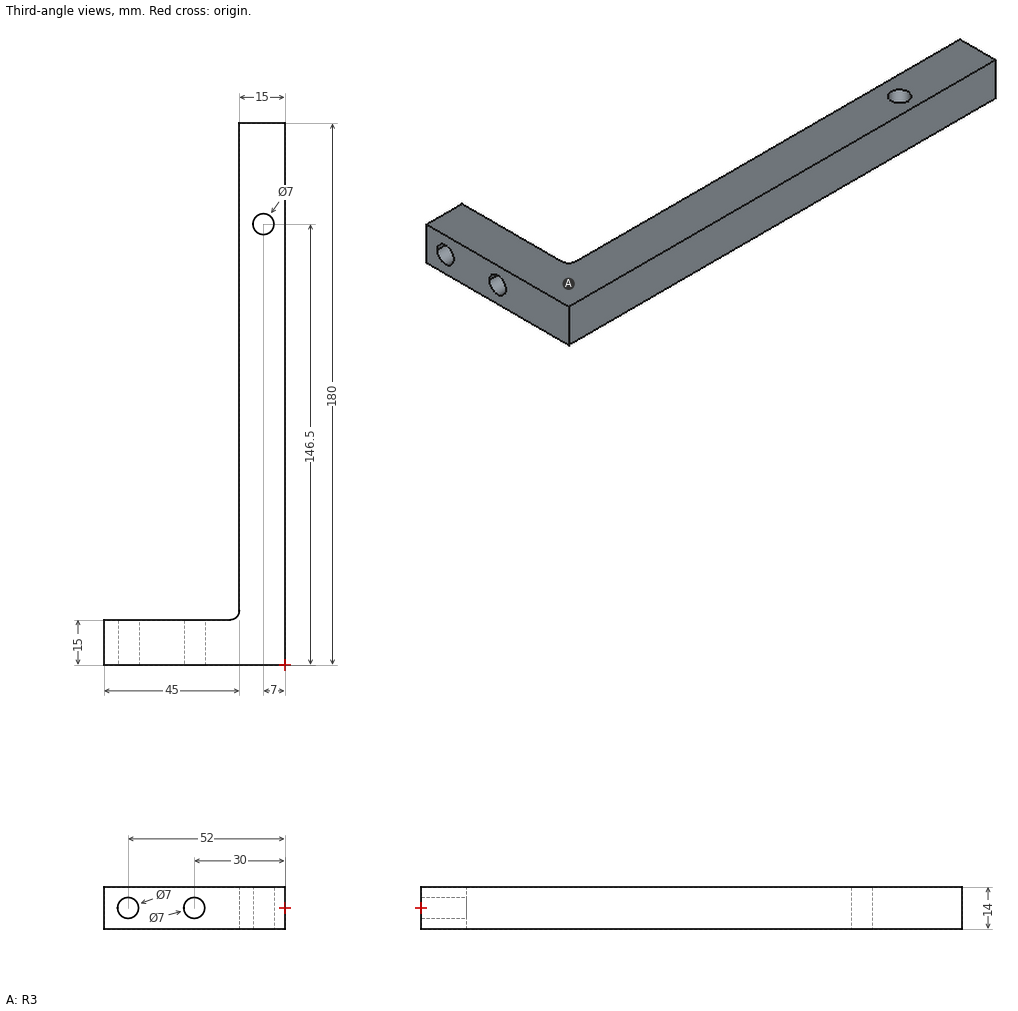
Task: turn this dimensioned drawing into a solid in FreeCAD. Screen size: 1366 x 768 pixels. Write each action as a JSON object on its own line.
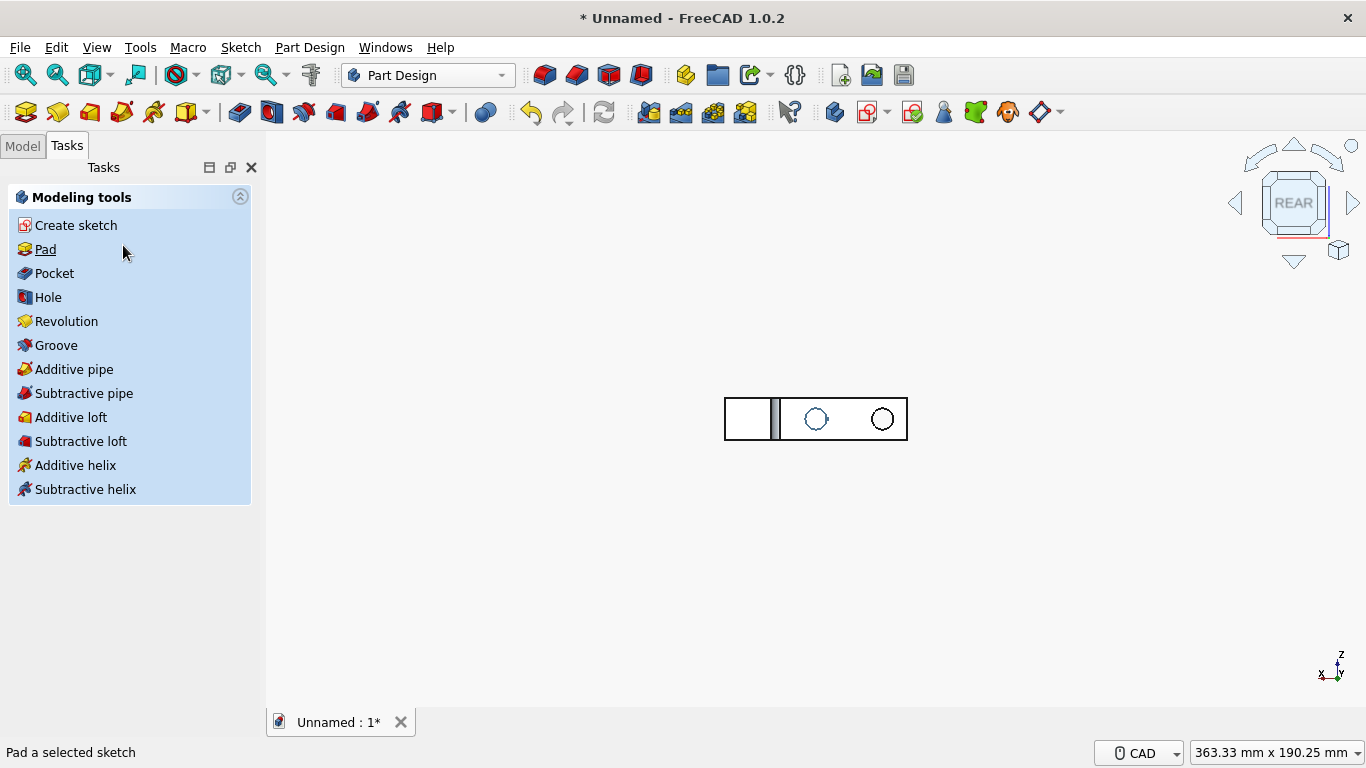
{"action": "left_click", "coordinate": [240, 112]}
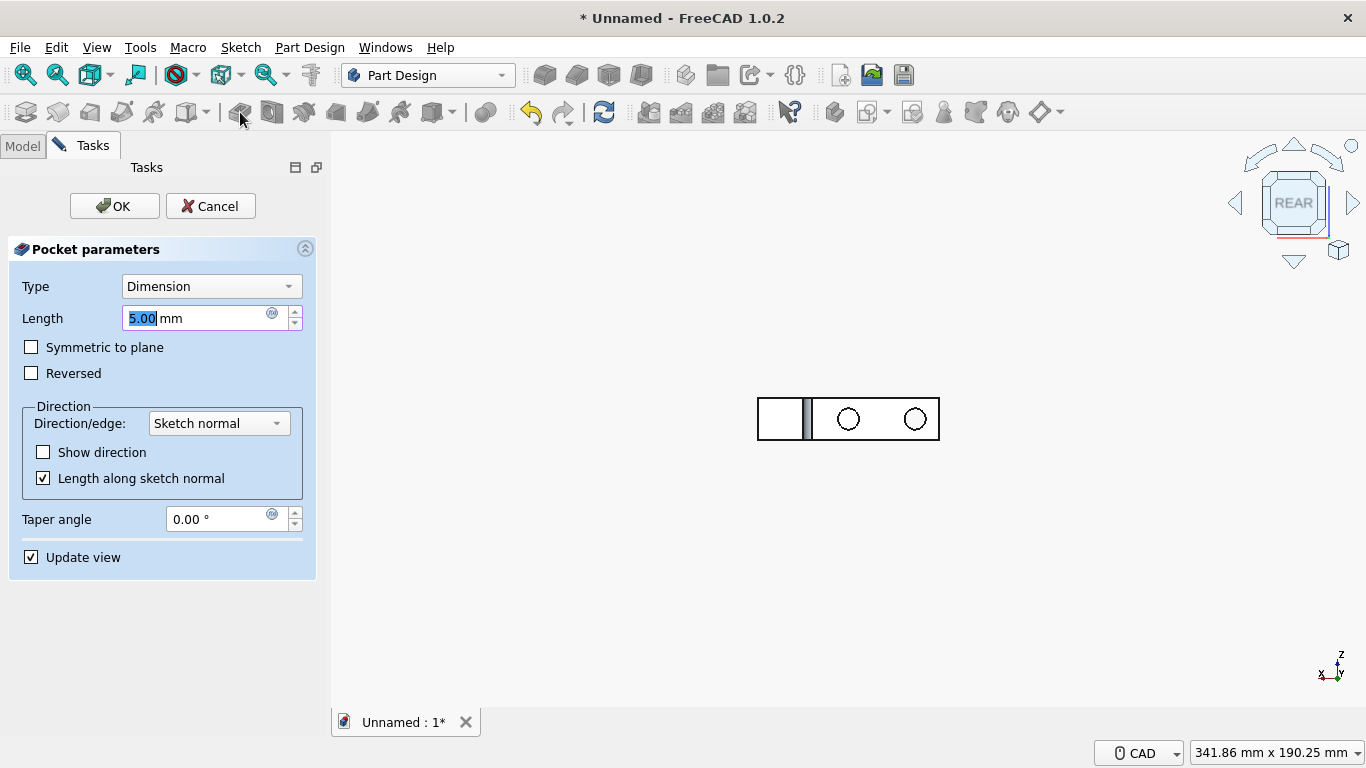
{"action": "left_click", "coordinate": [212, 286]}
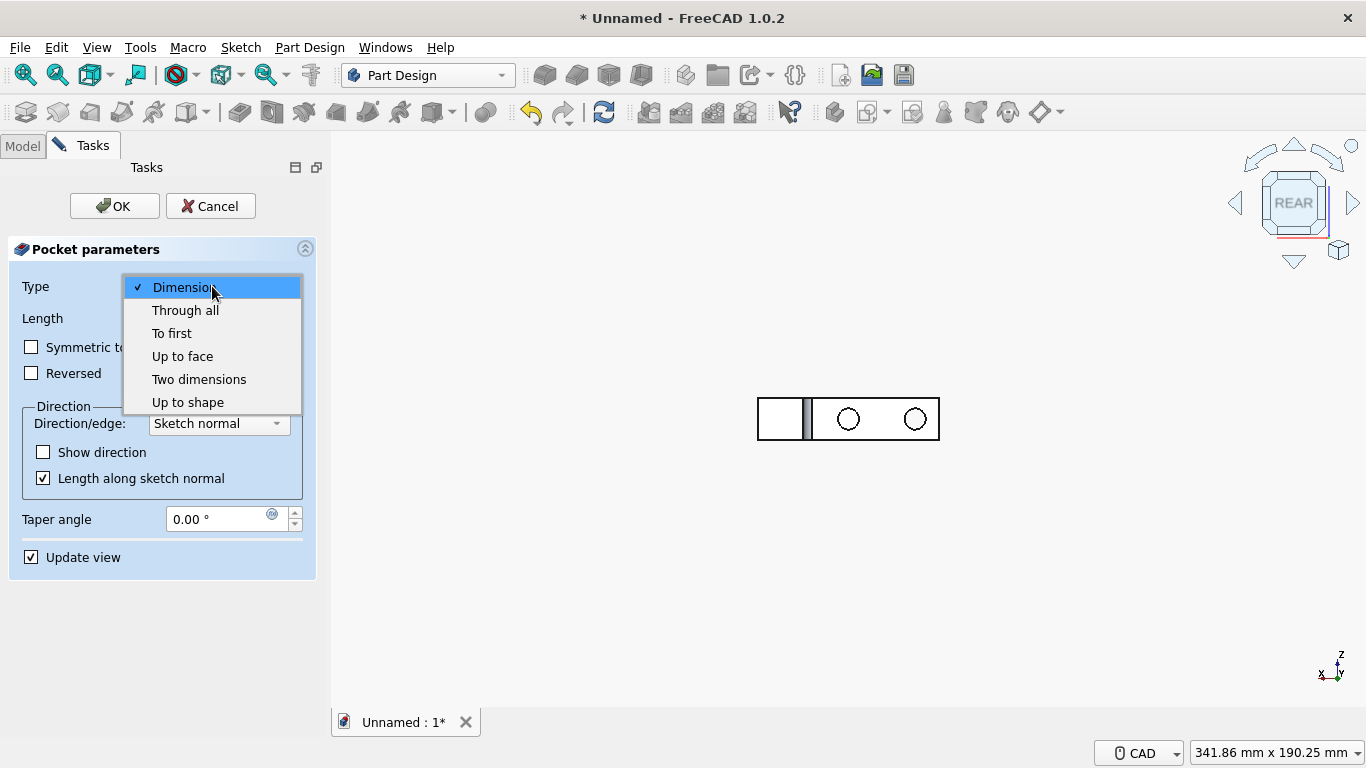
{"action": "left_click", "coordinate": [212, 334]}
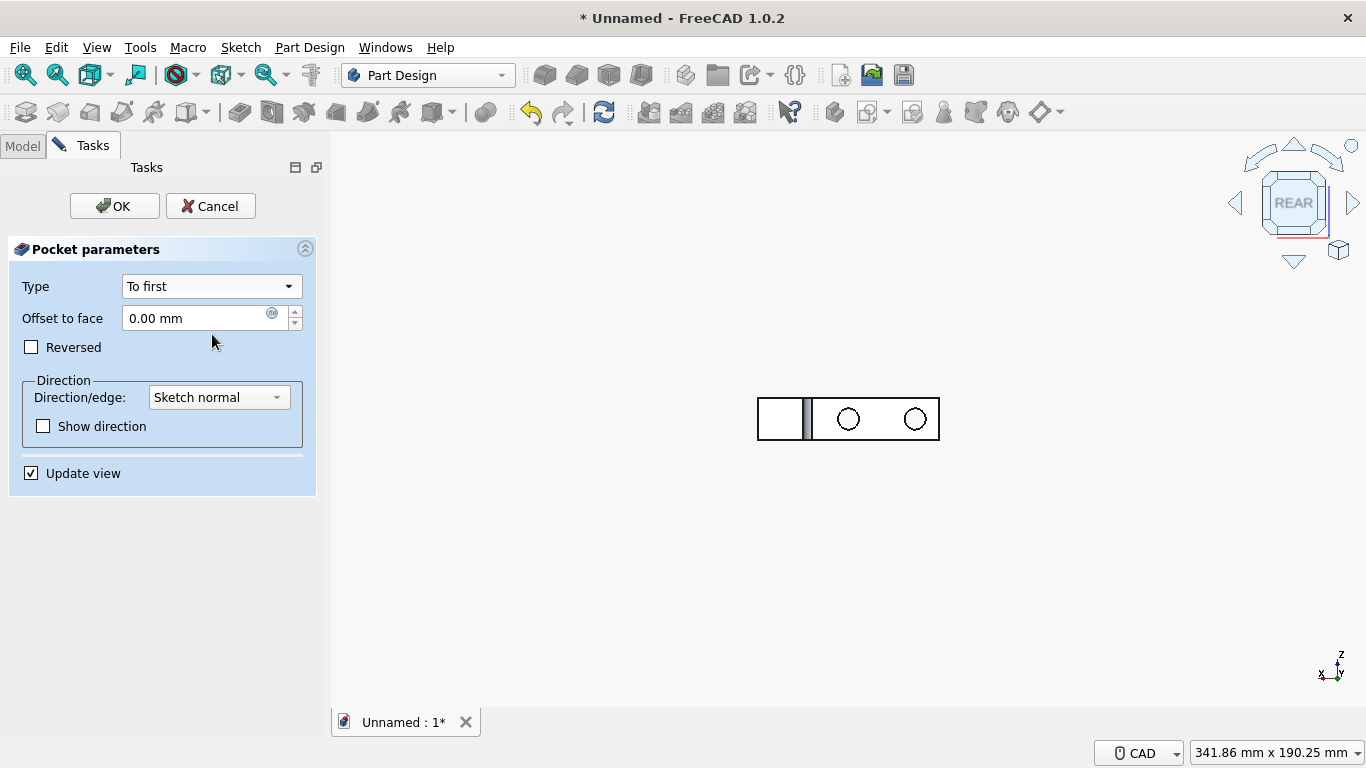
{"action": "left_click", "coordinate": [115, 206]}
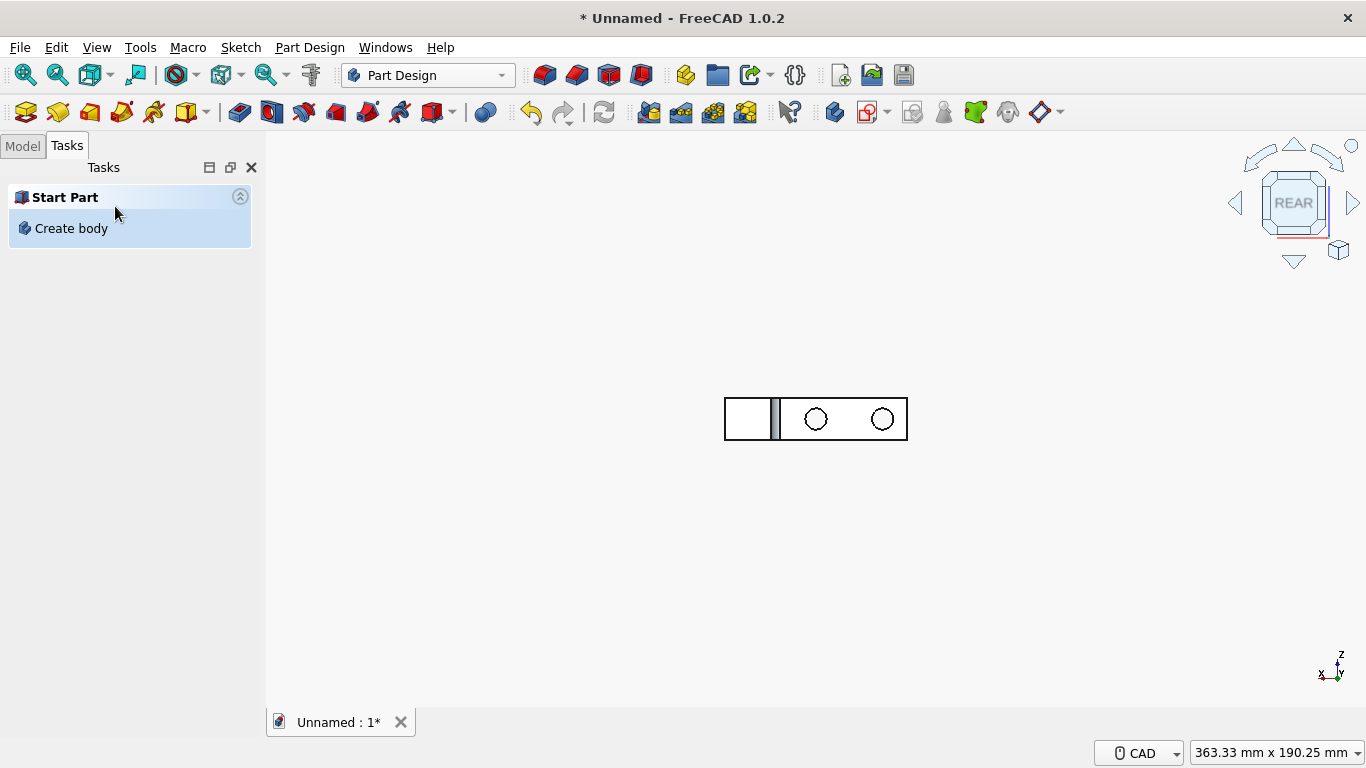
{"action": "left_click", "coordinate": [26, 76]}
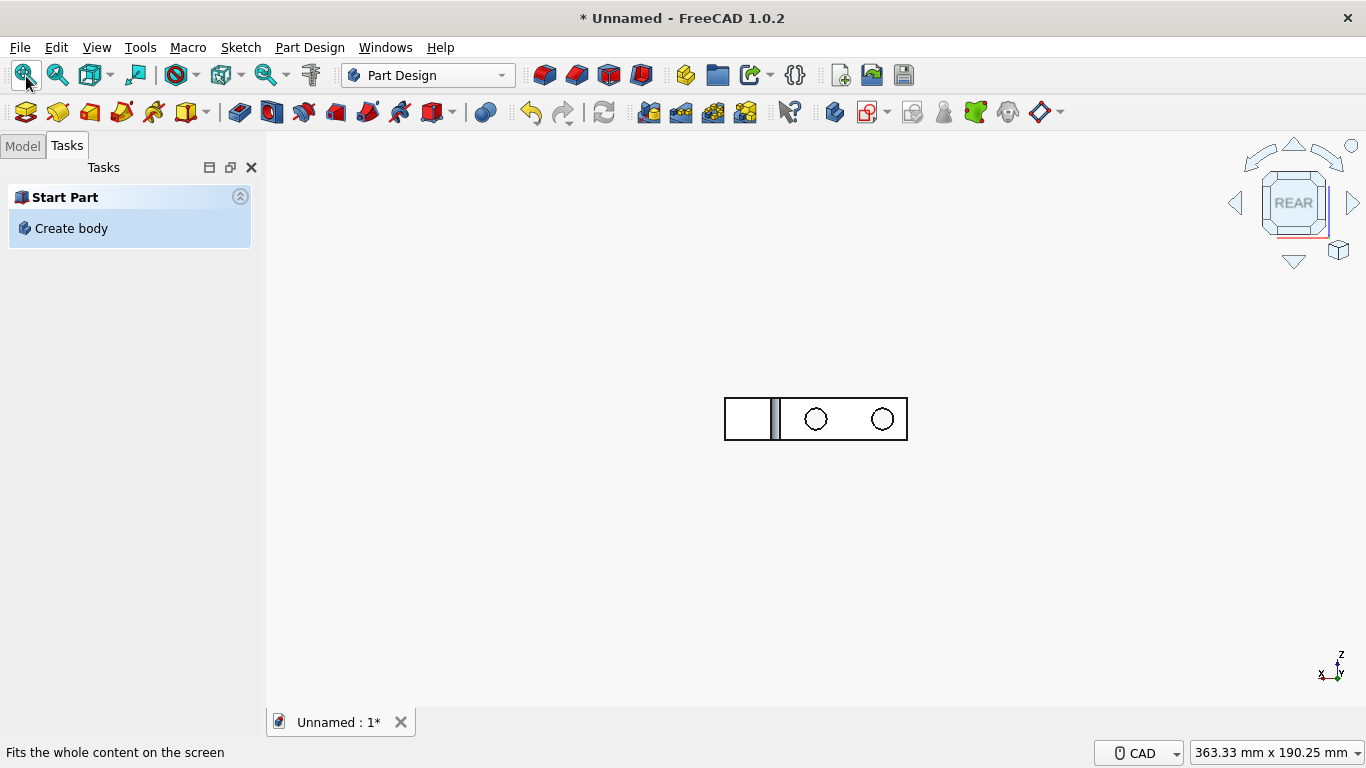
{"action": "key", "text": "5"}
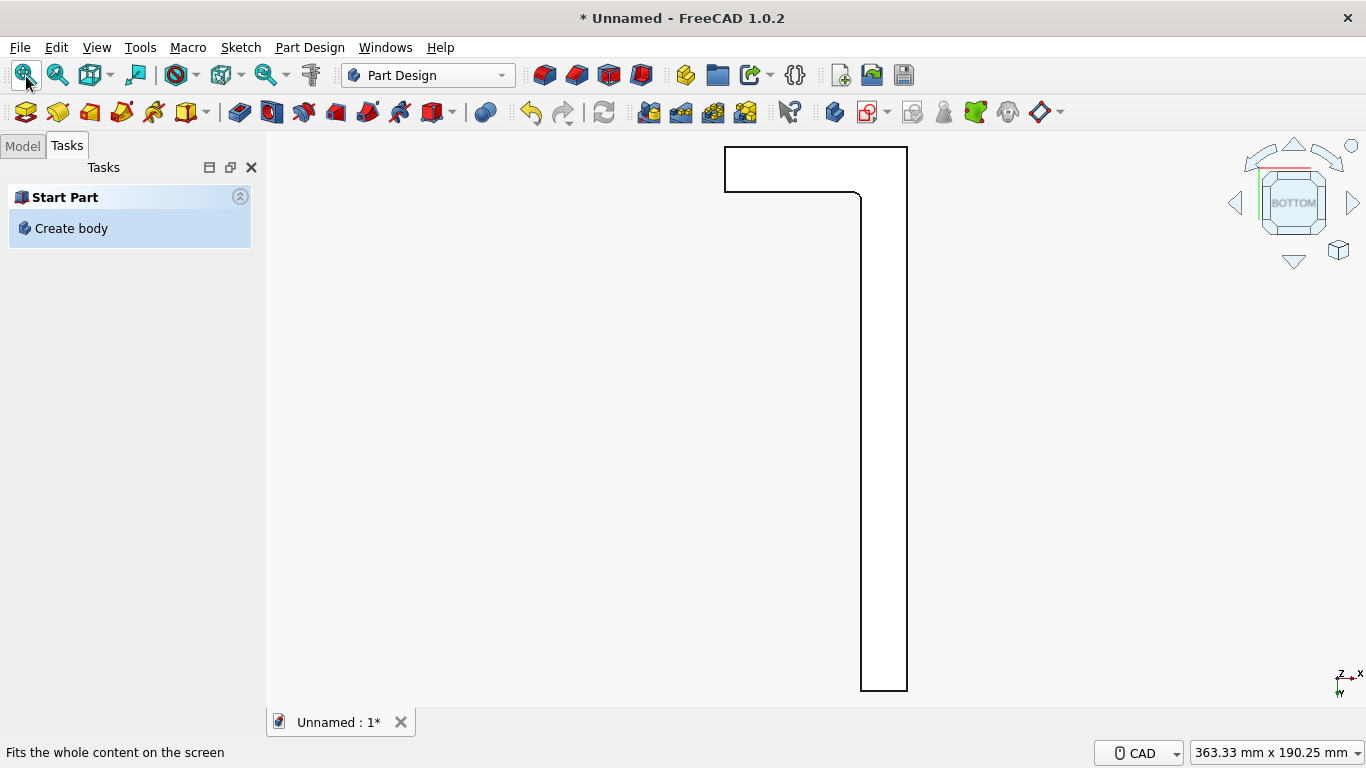
{"action": "left_click", "coordinate": [894, 652]}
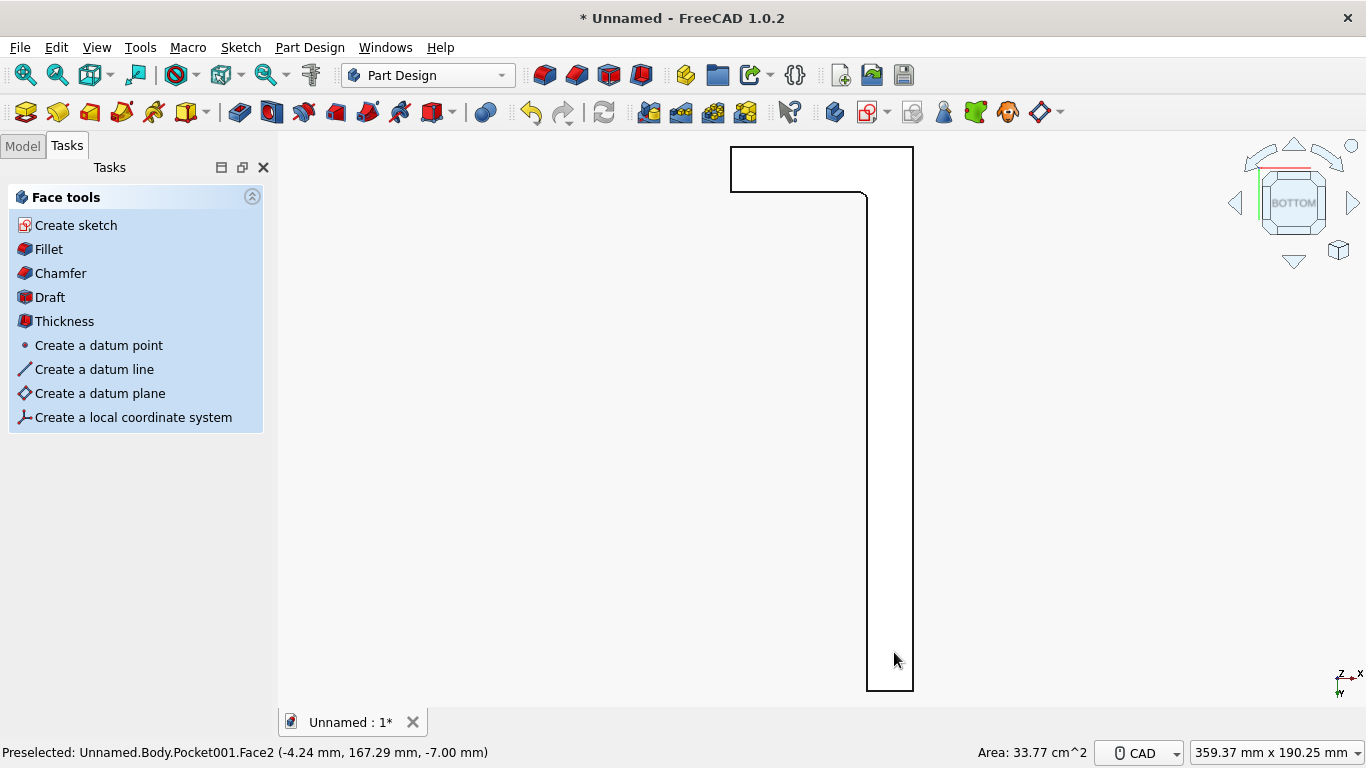
{"action": "left_click", "coordinate": [868, 112]}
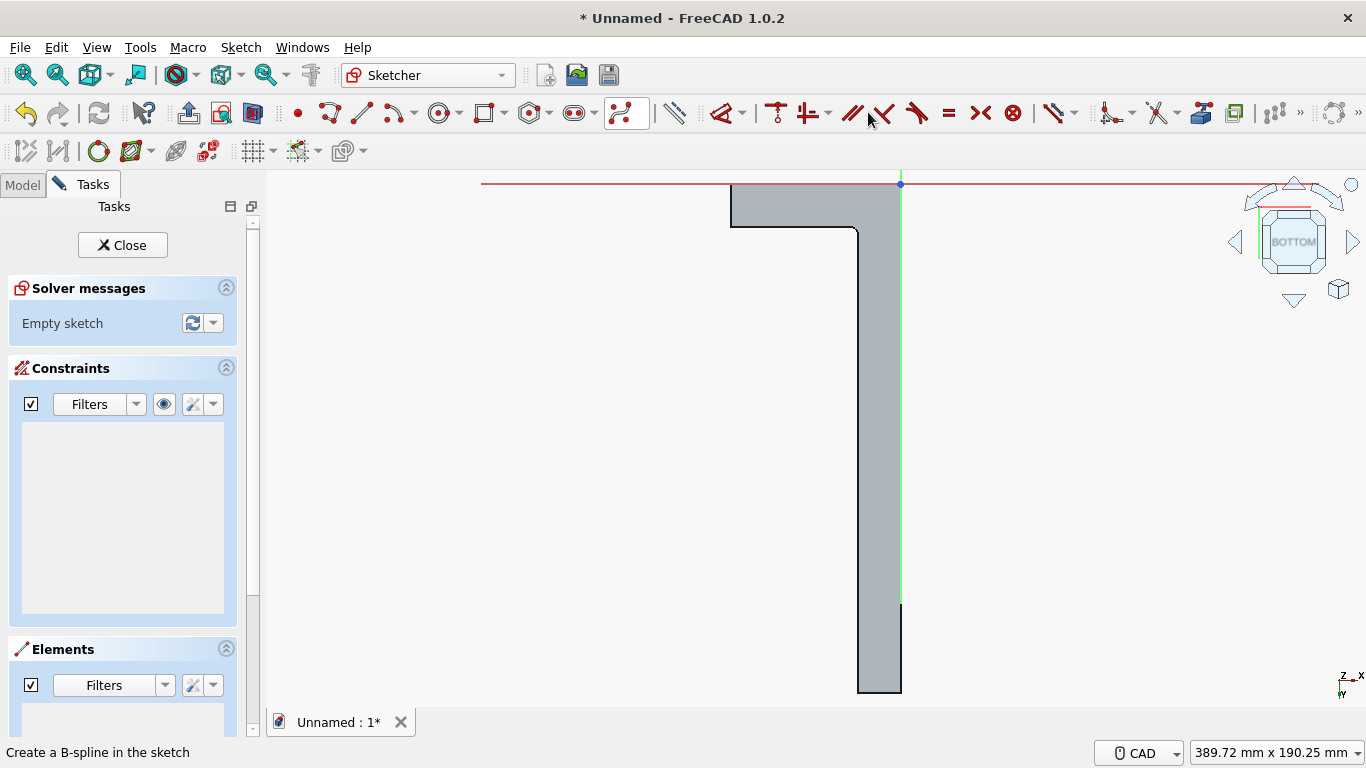
{"action": "scroll", "coordinate": [890, 608], "scroll_direction": "up", "scroll_amount": 14}